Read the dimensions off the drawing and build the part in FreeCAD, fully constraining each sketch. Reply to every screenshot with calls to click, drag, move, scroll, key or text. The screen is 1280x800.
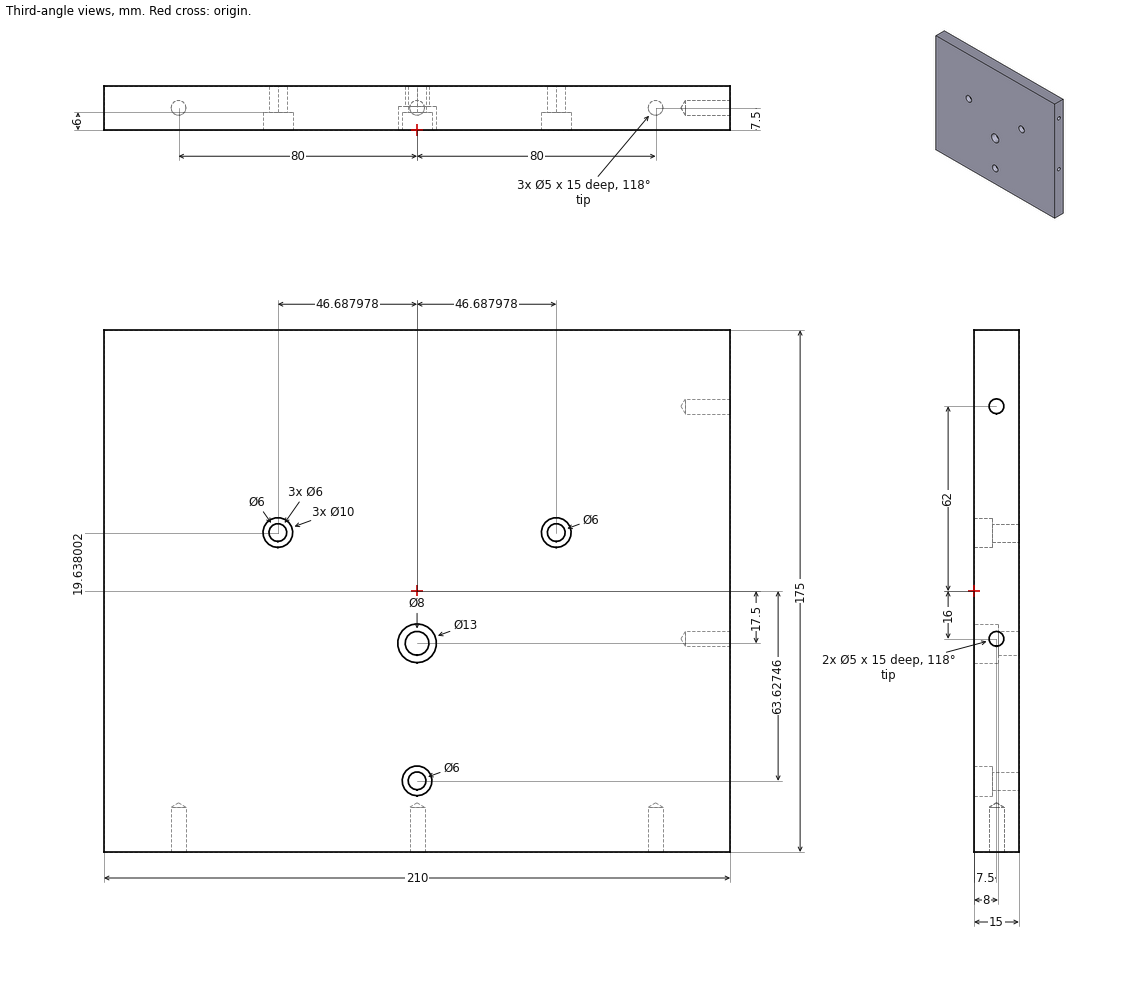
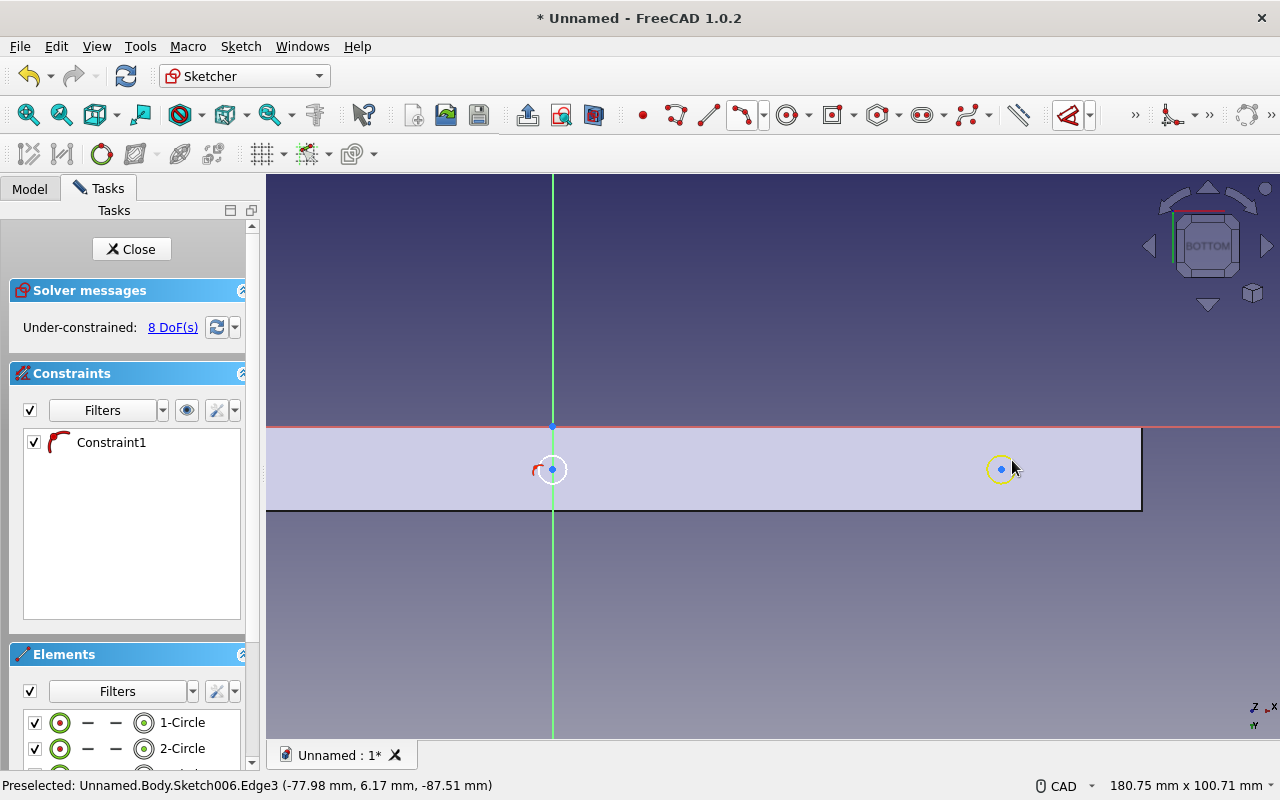
click(1011, 460)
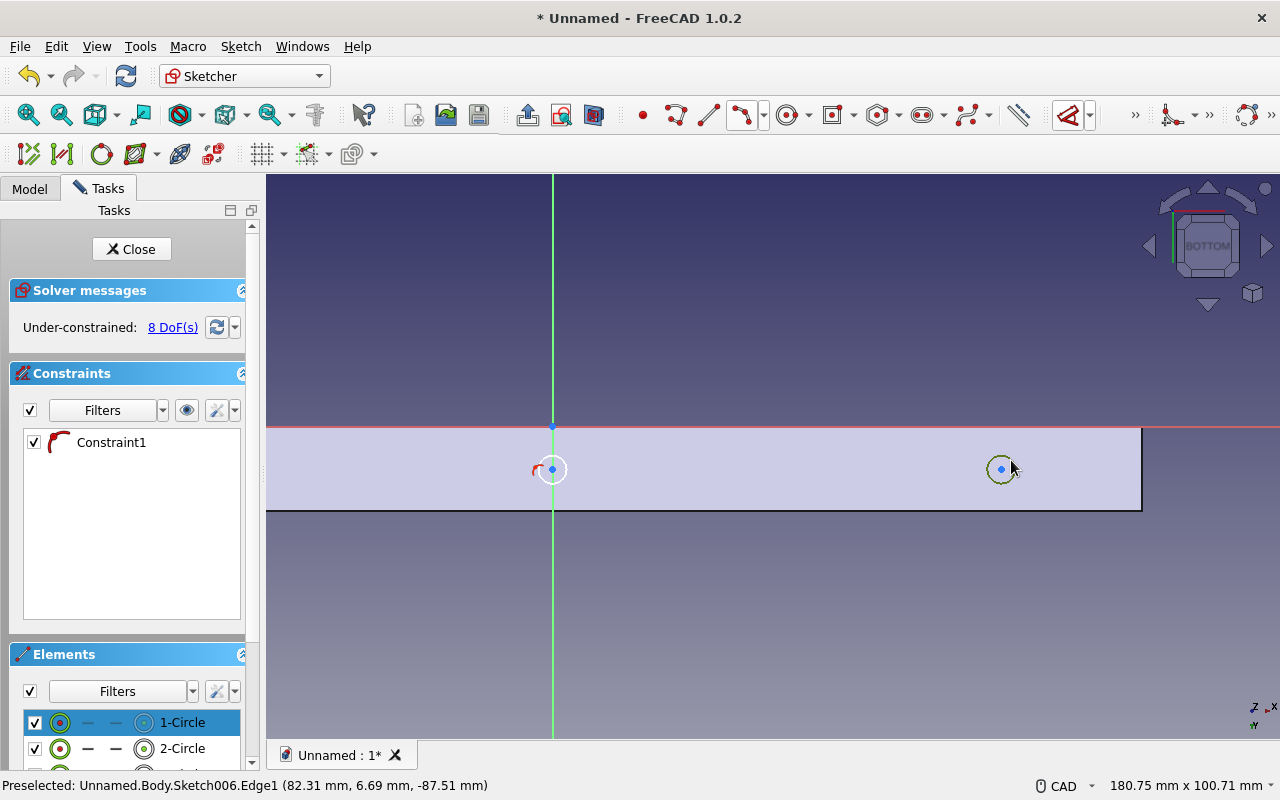
scroll(562, 460, up, 2)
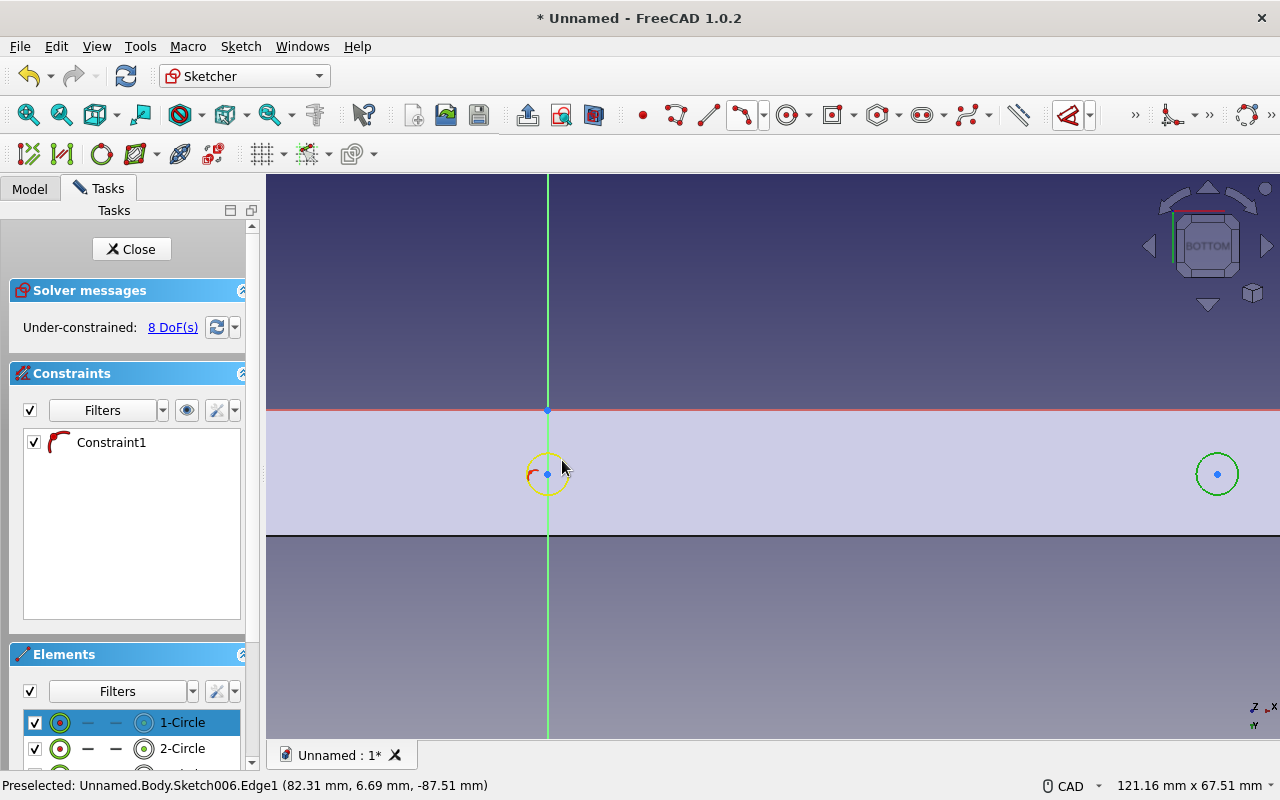
click(562, 460)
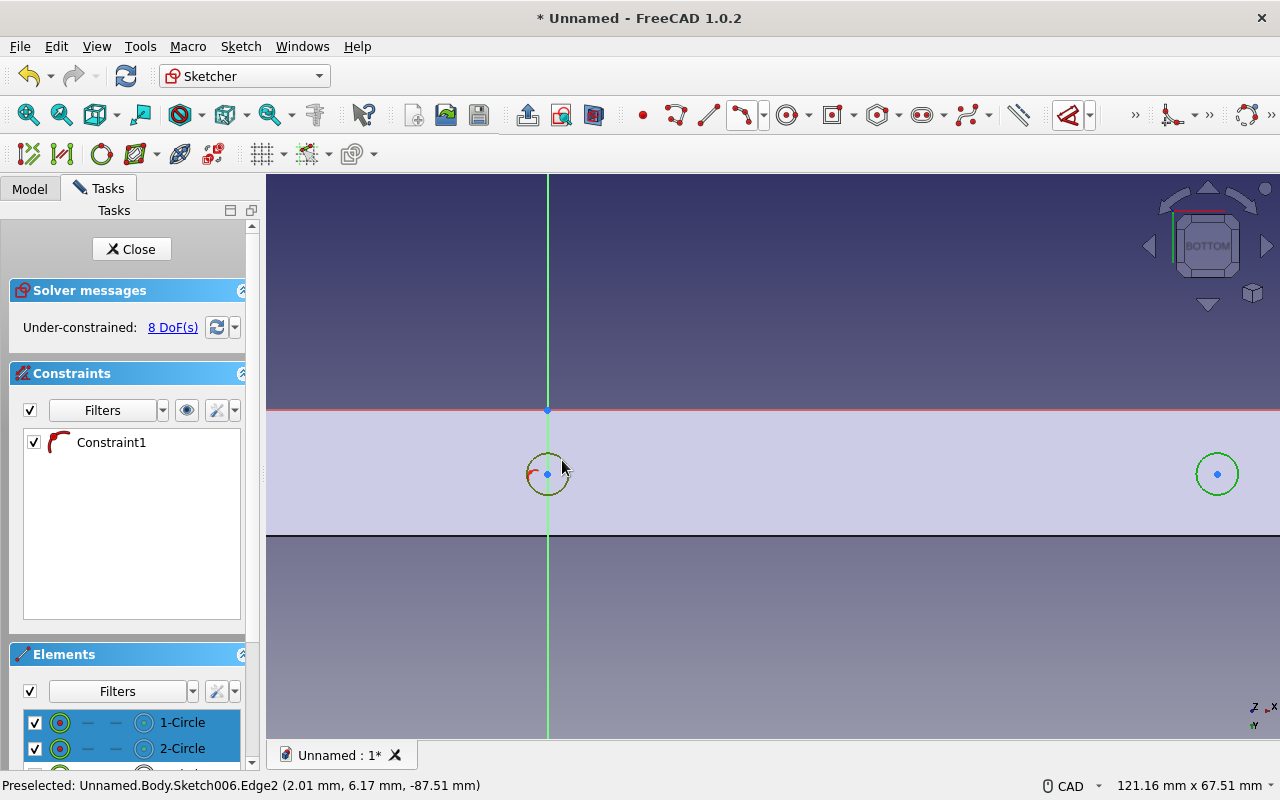
scroll(832, 460, down, 4)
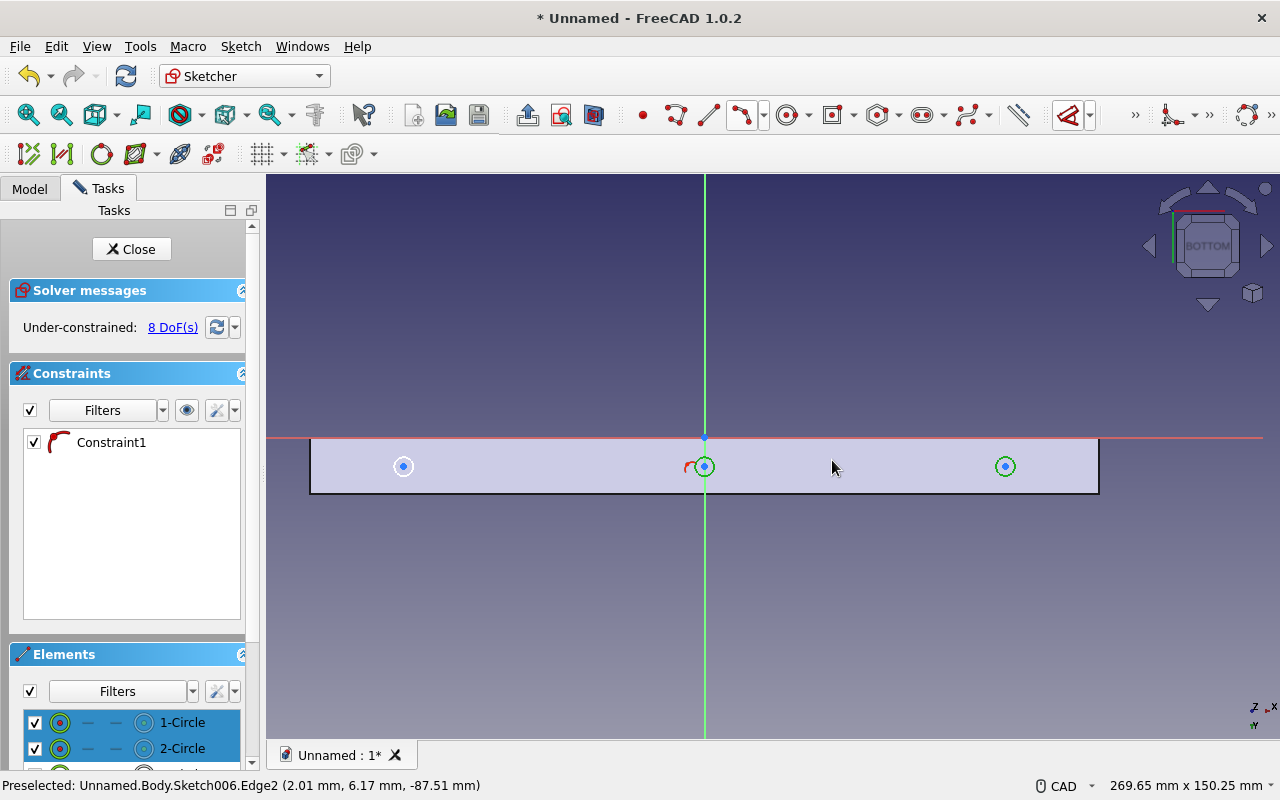
scroll(410, 460, up, 2)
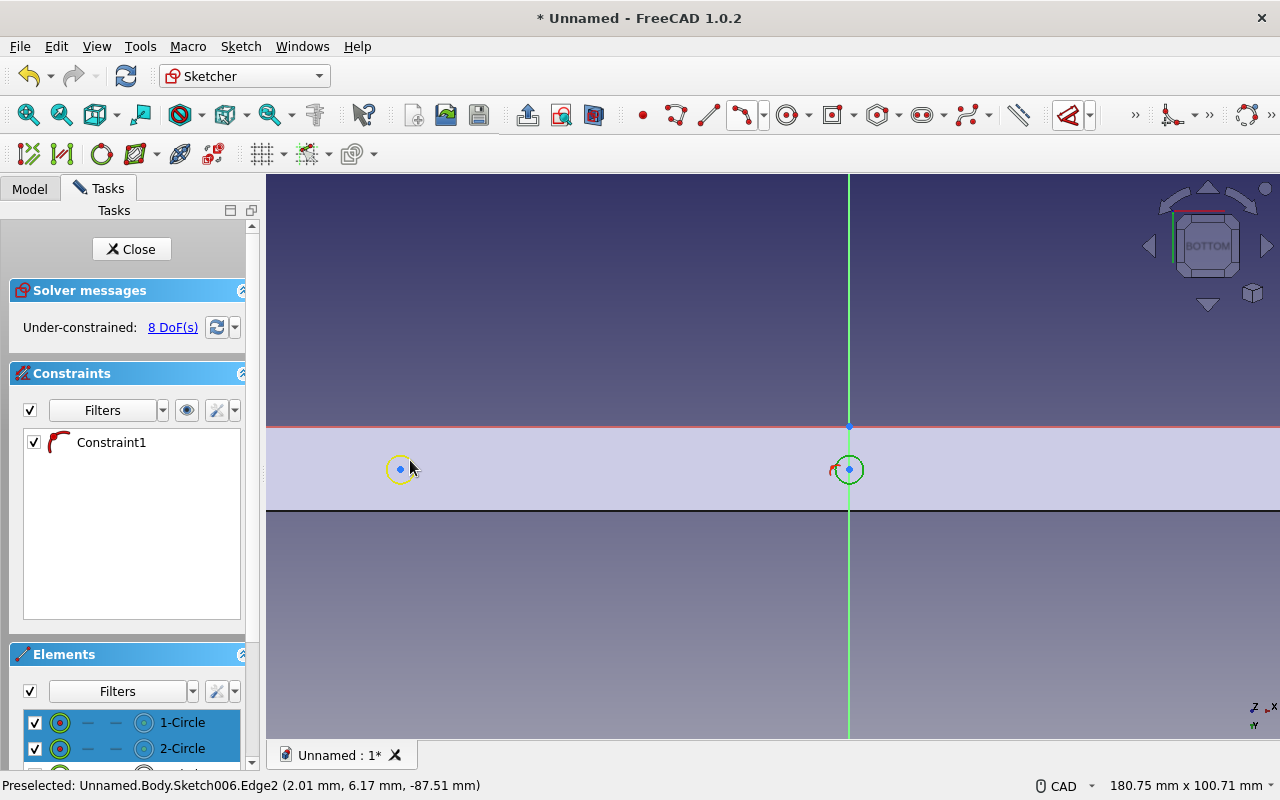
click(410, 460)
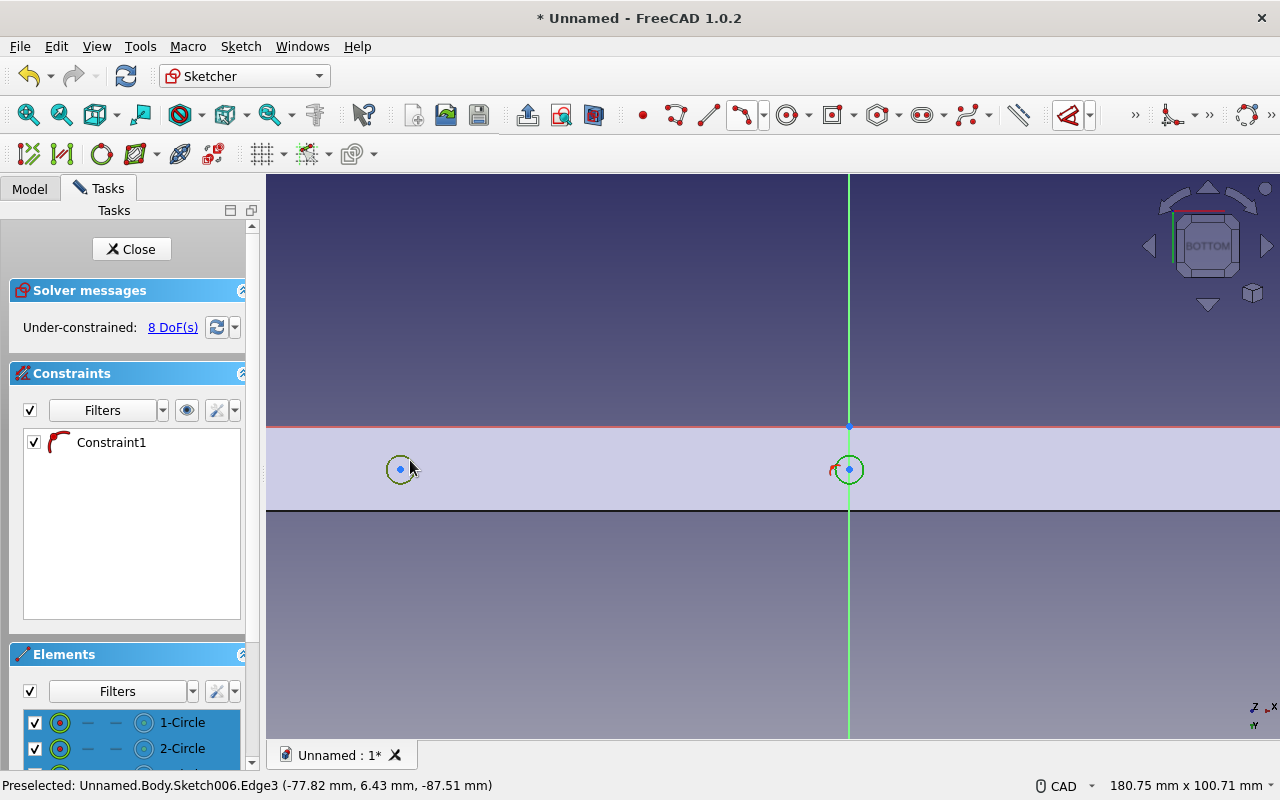
key(e)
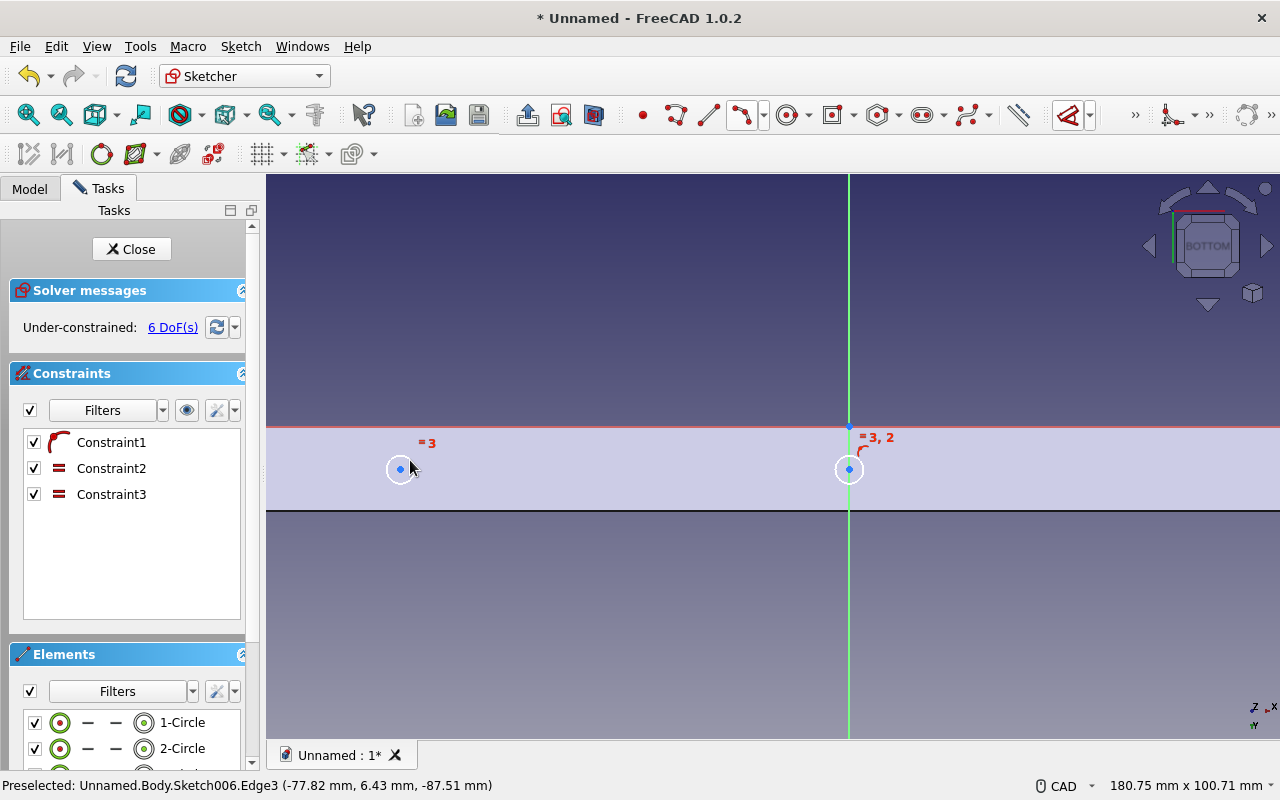
scroll(410, 460, down, 2)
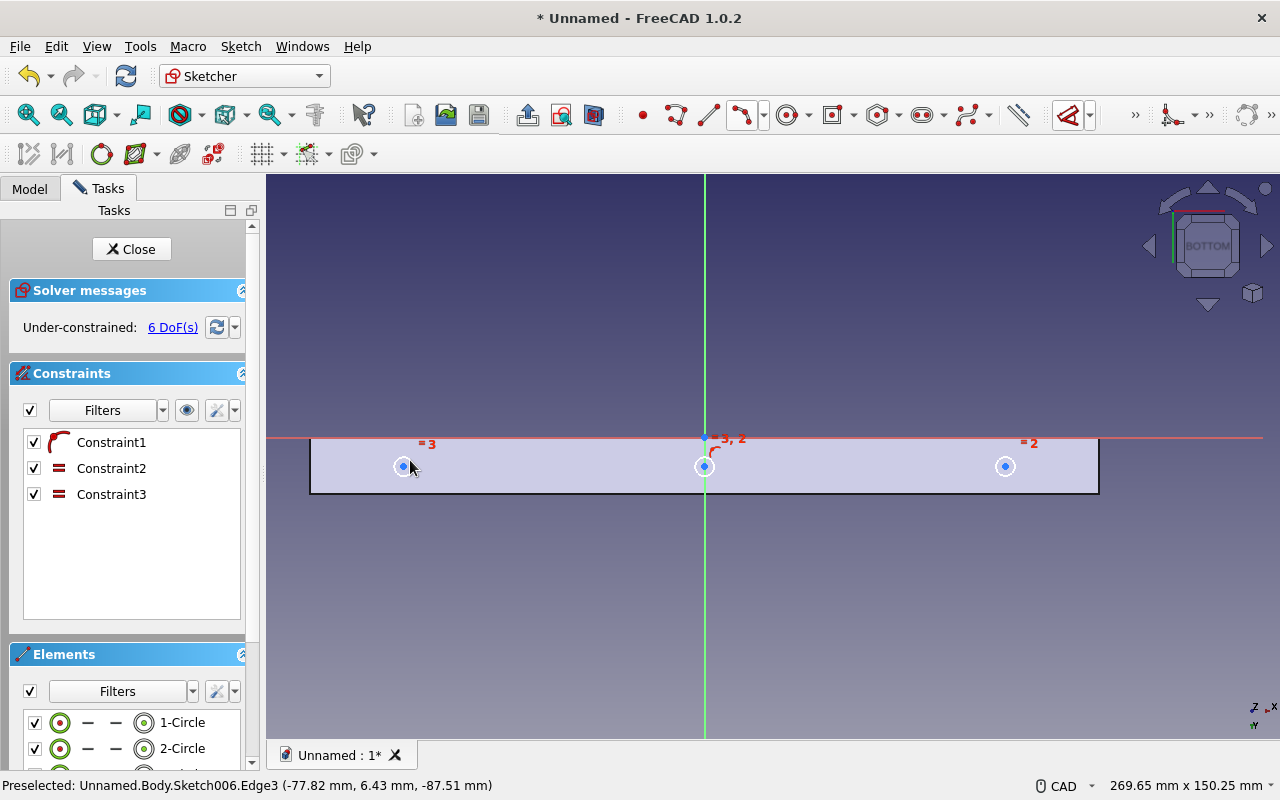
click(1005, 467)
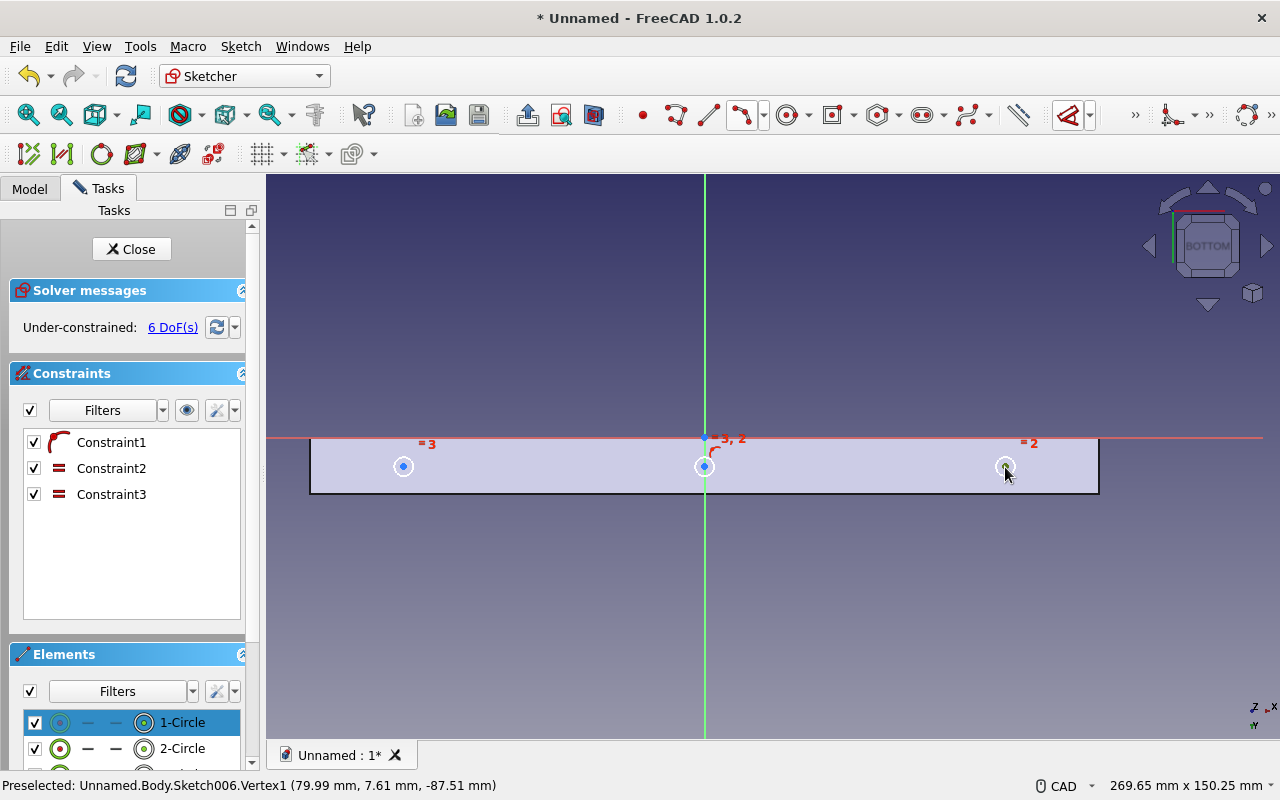
click(705, 467)